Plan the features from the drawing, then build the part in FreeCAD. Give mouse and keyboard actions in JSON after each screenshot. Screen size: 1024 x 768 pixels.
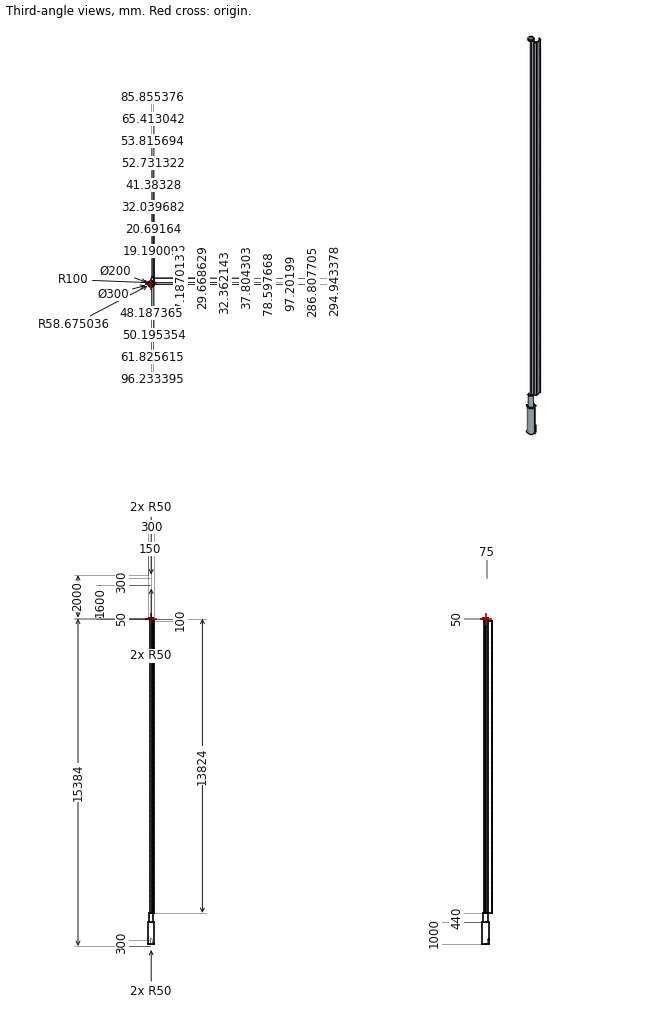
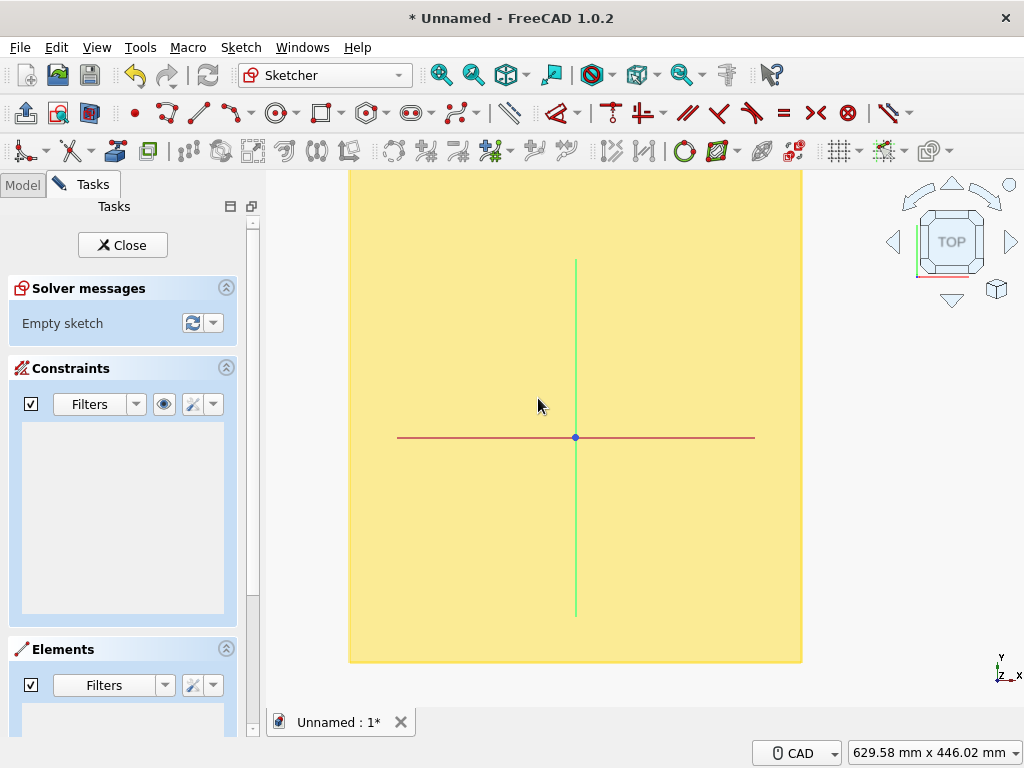
{"action": "left_click", "coordinate": [276, 114]}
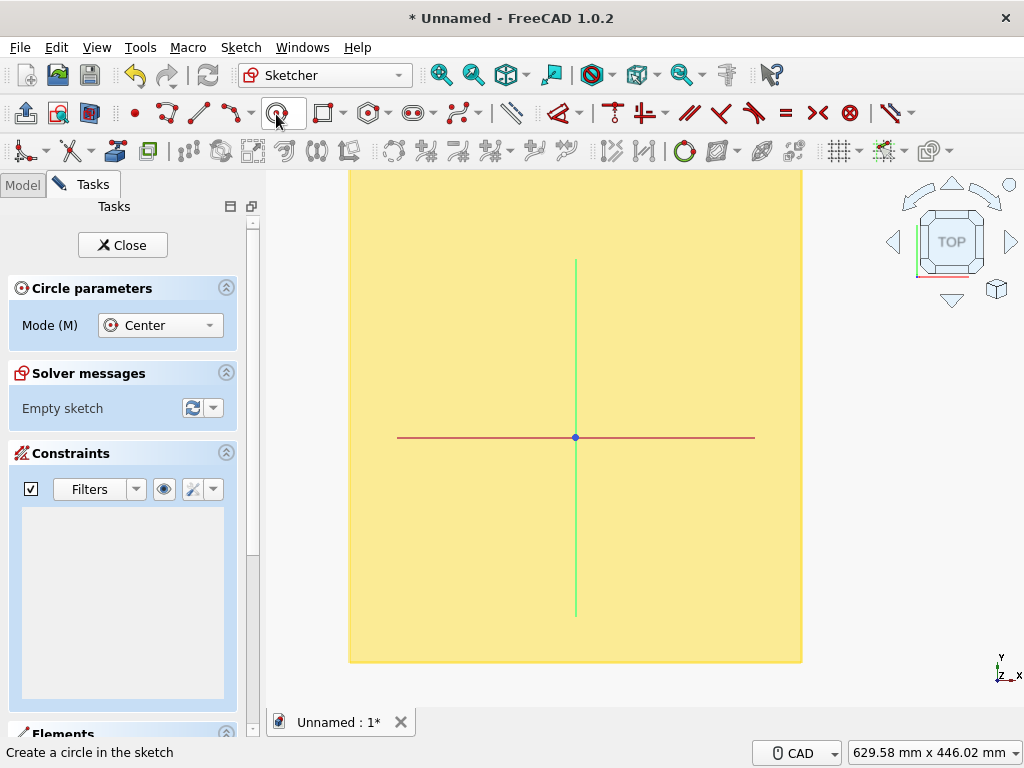
{"action": "left_click", "coordinate": [576, 438]}
{"action": "left_click", "coordinate": [704, 310]}
{"action": "key", "text": "Escape"}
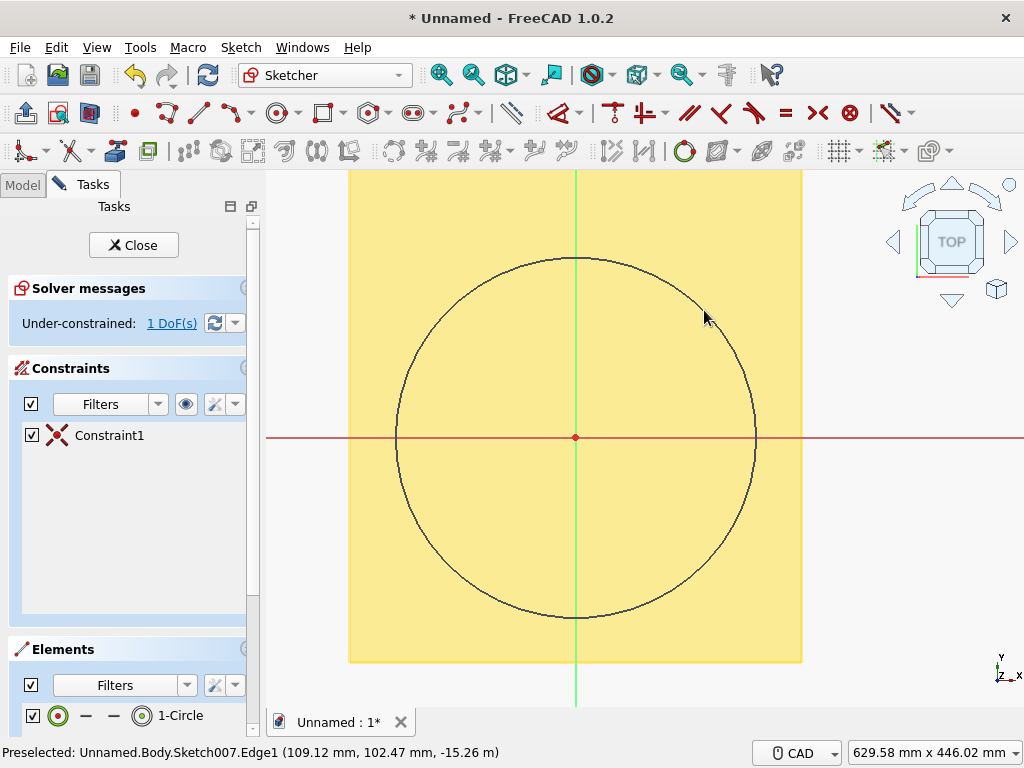
{"action": "left_click", "coordinate": [558, 114]}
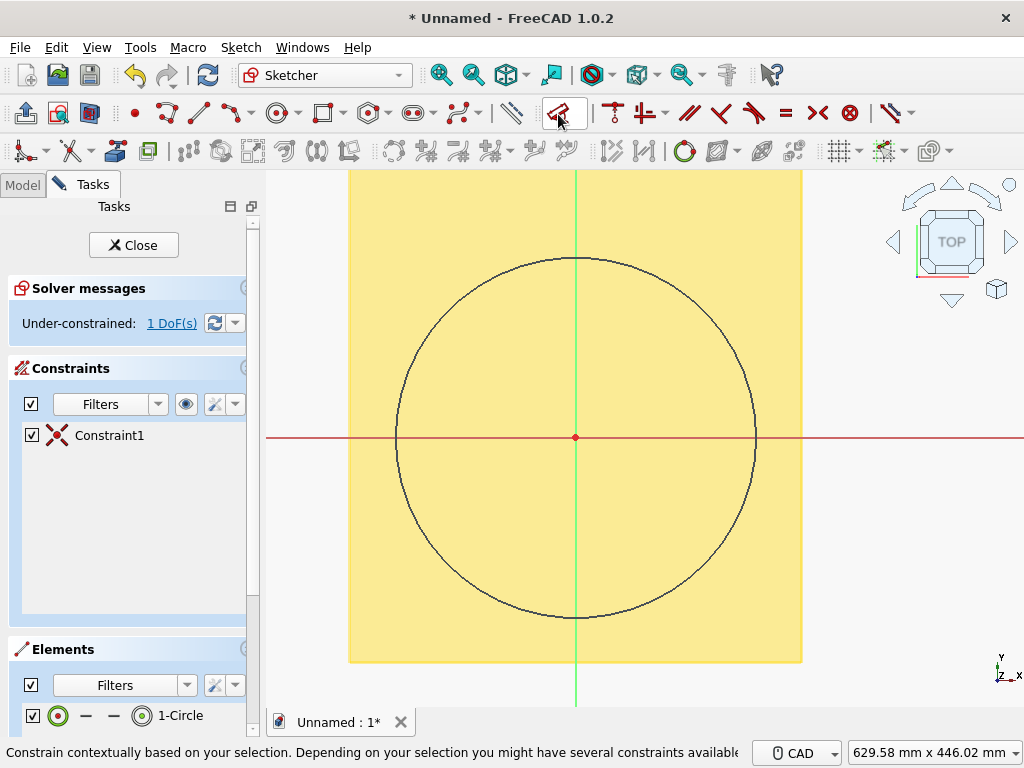
{"action": "left_click", "coordinate": [703, 310]}
{"action": "left_click", "coordinate": [726, 287]}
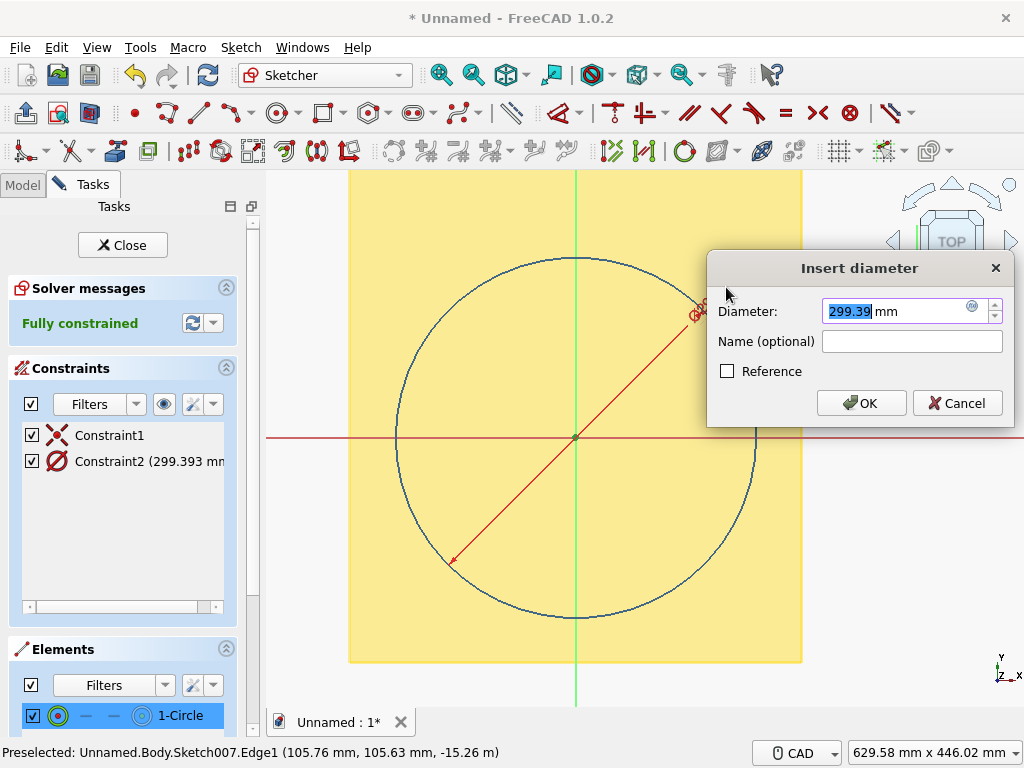
{"action": "type", "text": "300"}
{"action": "key", "text": "Return"}
{"action": "key", "text": "Escape"}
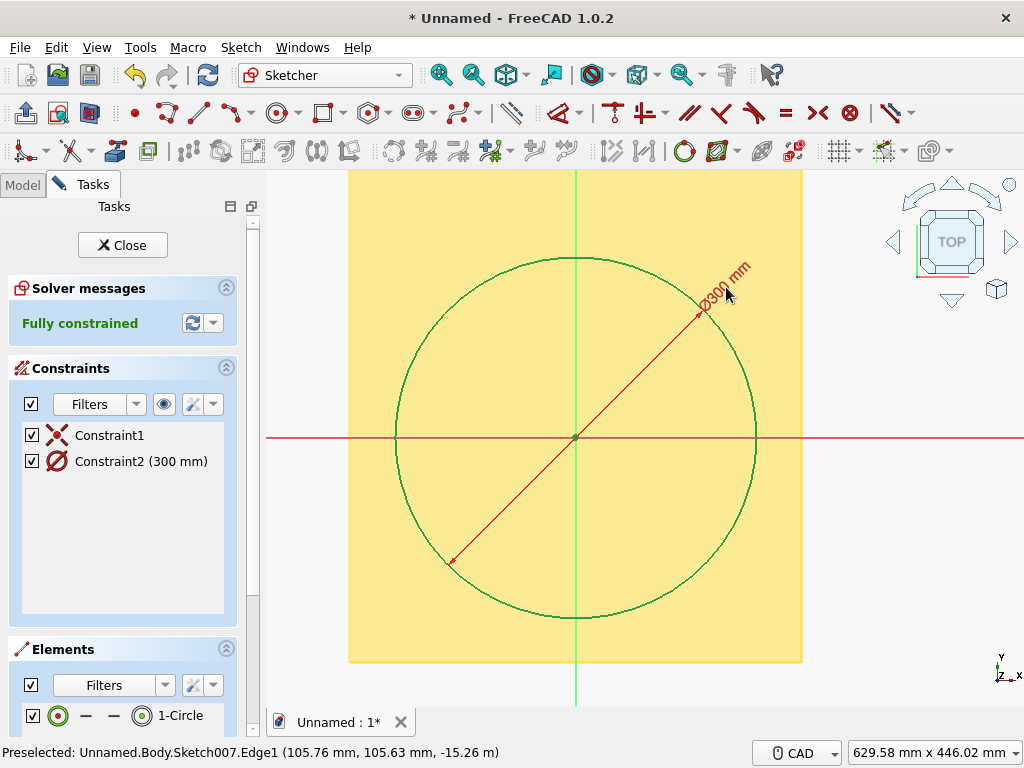
{"action": "left_click", "coordinate": [123, 245]}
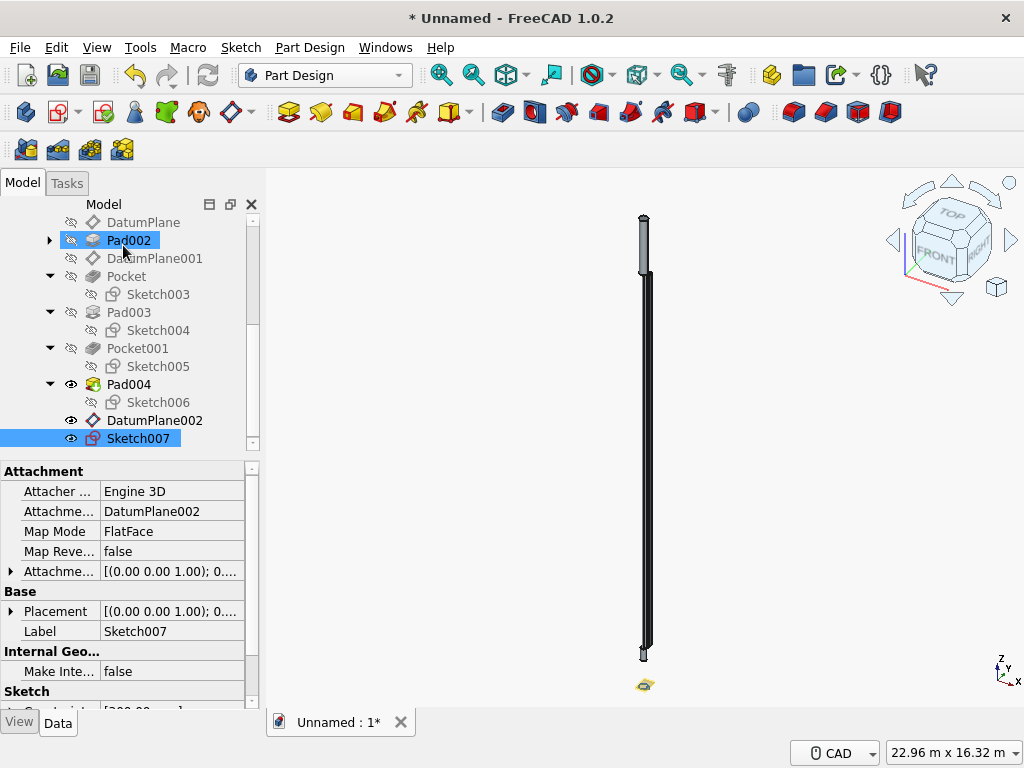
{"action": "left_click", "coordinate": [290, 112]}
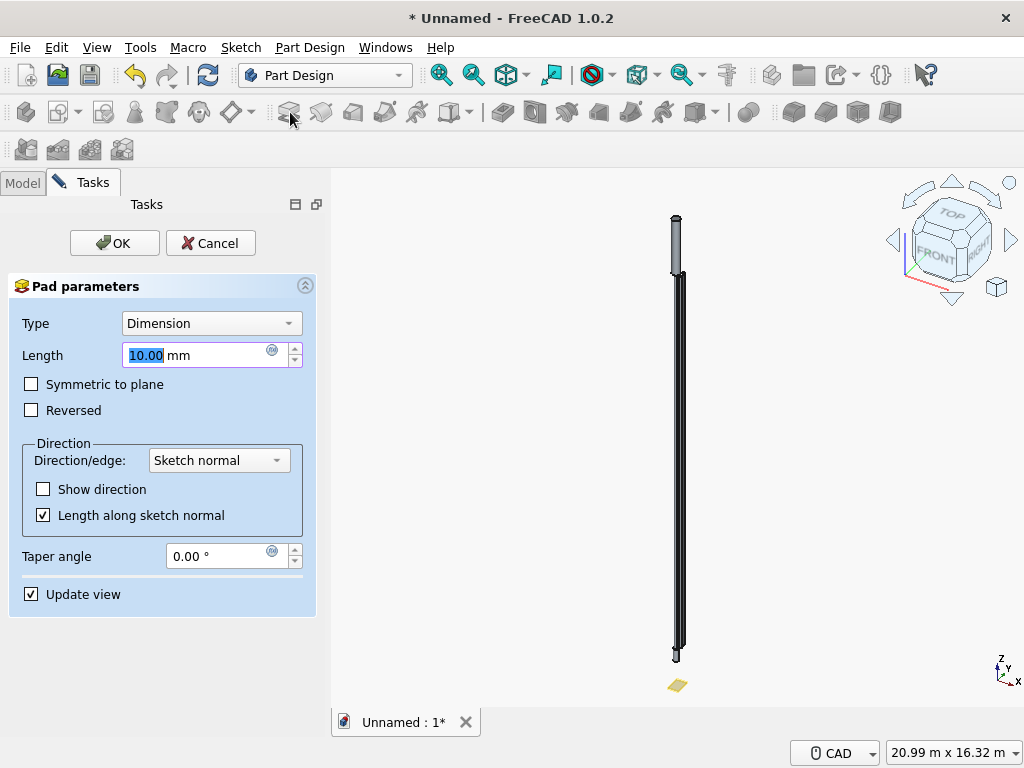
{"action": "type", "text": "1000"}
{"action": "key", "text": "Tab"}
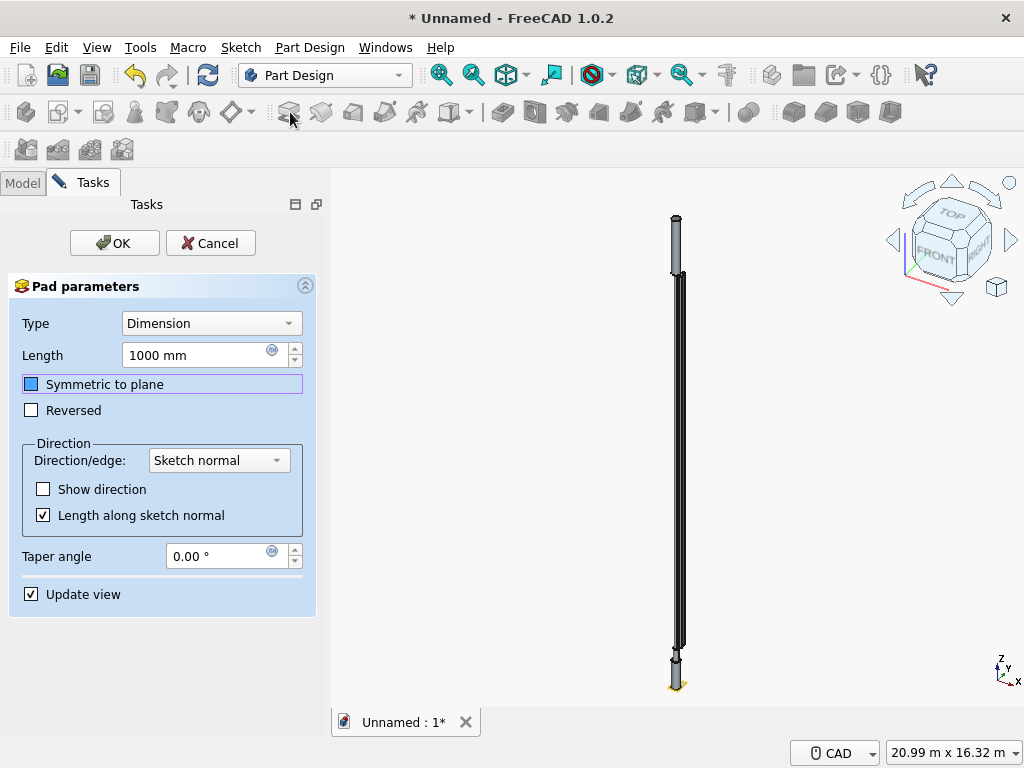
{"action": "left_click", "coordinate": [115, 243]}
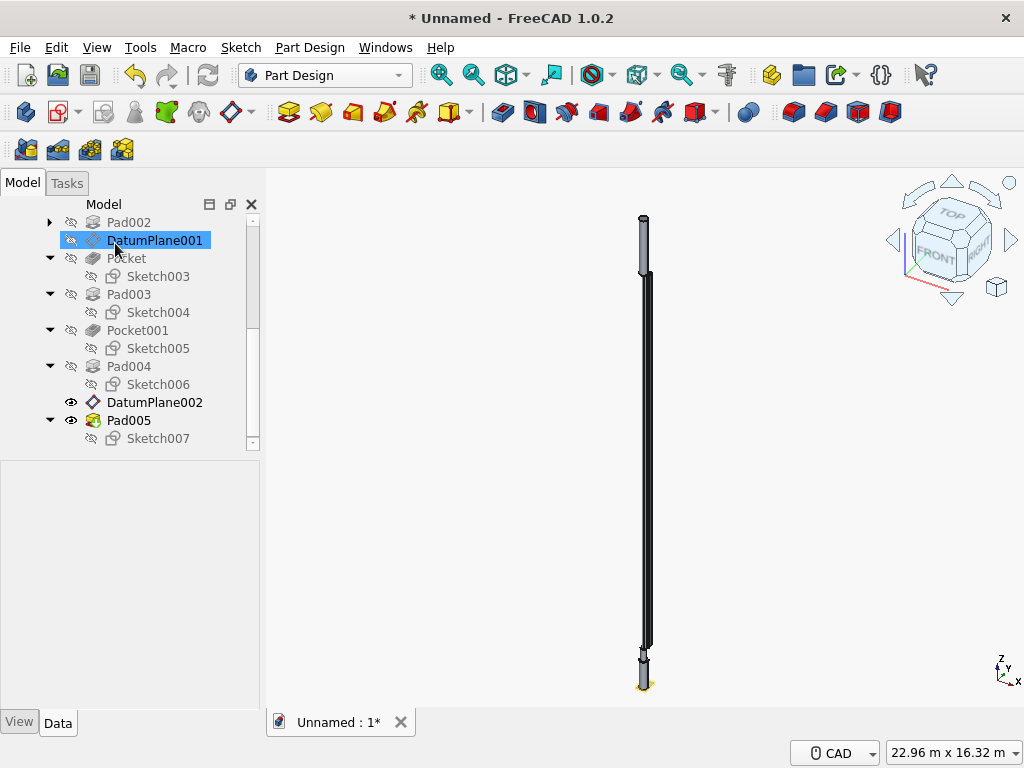
{"action": "left_click", "coordinate": [116, 402]}
{"action": "key", "text": "space"}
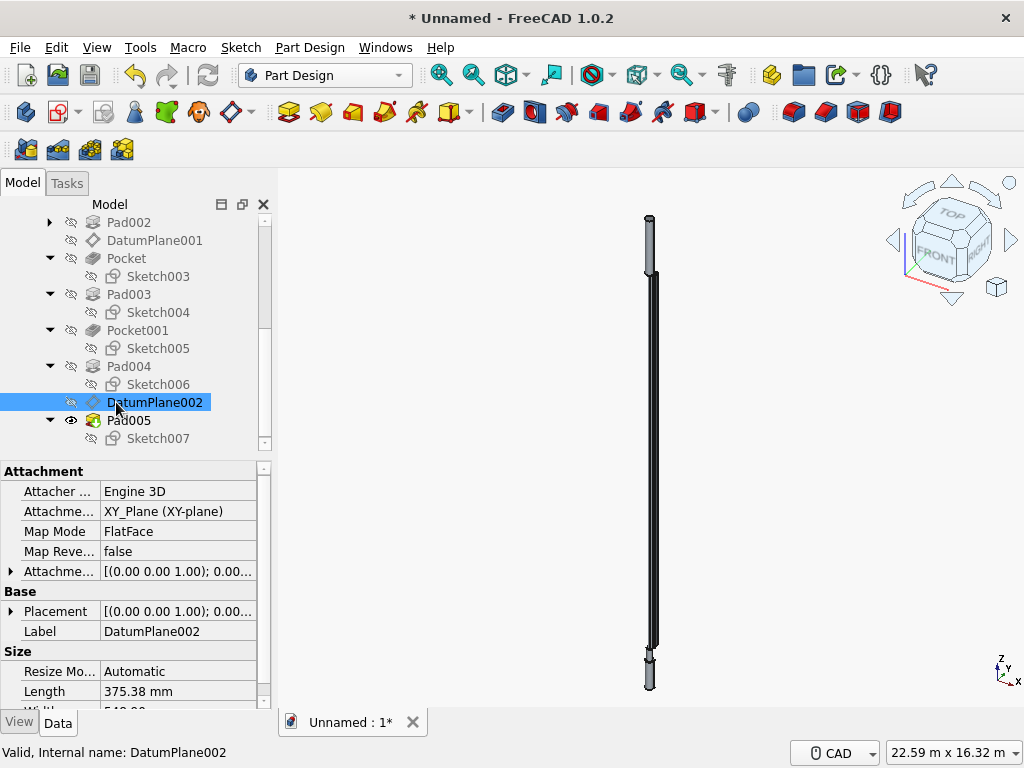
{"action": "scroll", "coordinate": [140, 326], "scroll_direction": "down", "scroll_amount": 3}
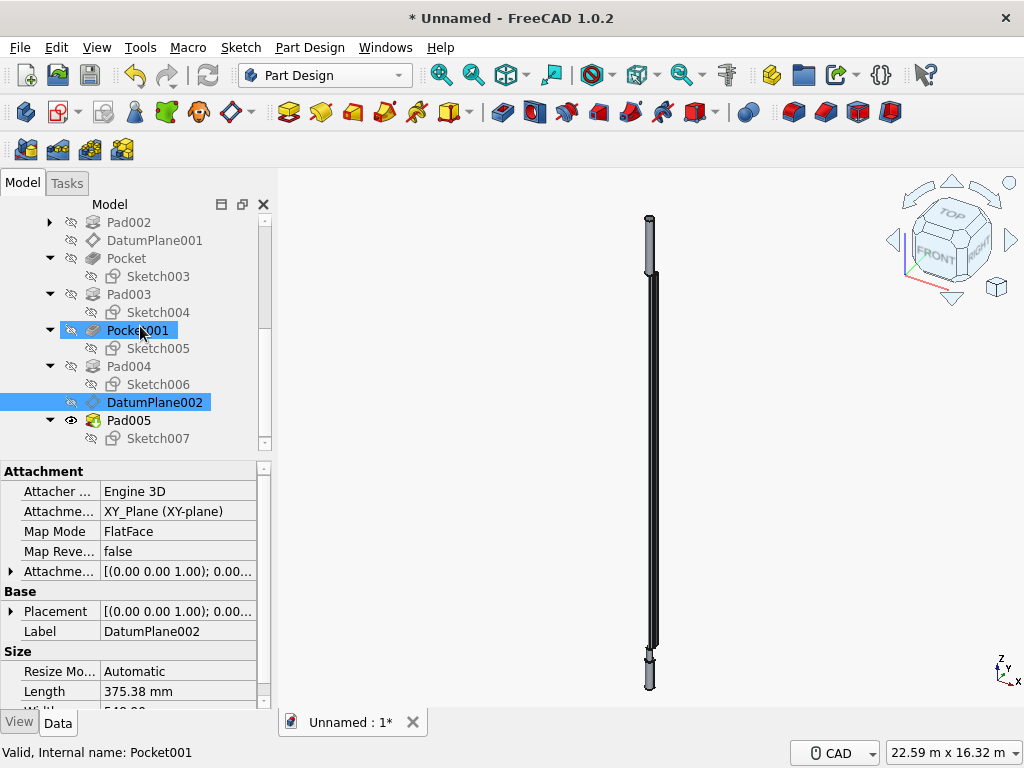
{"action": "scroll", "coordinate": [140, 326], "scroll_direction": "up", "scroll_amount": 15}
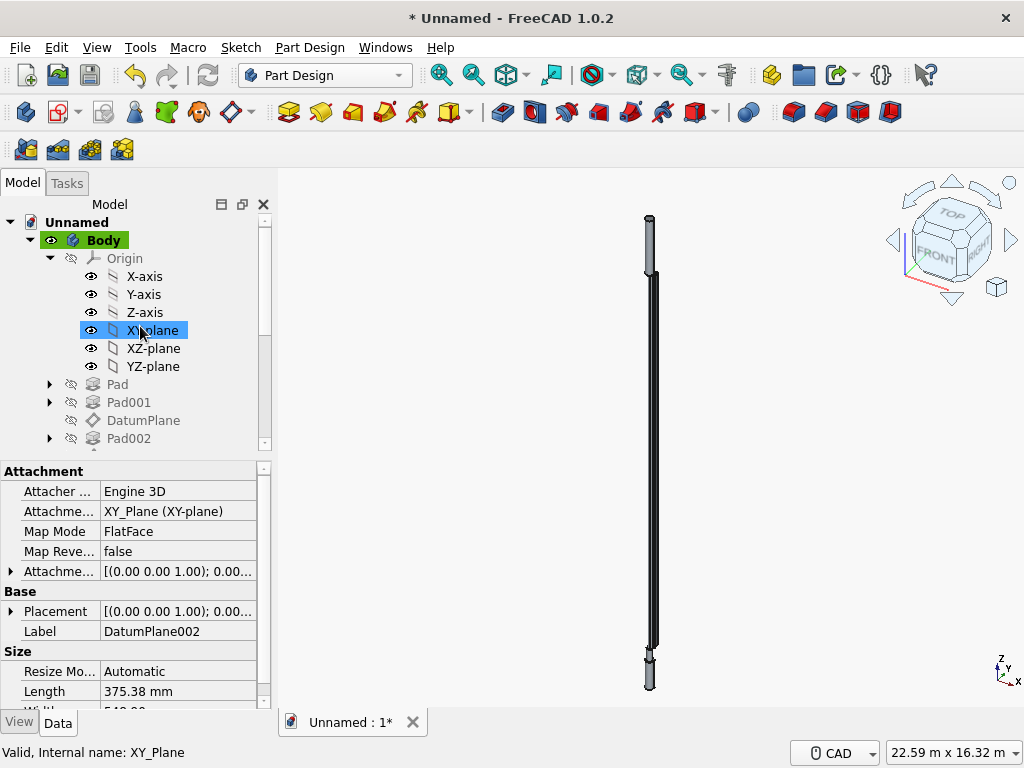
{"action": "left_click", "coordinate": [136, 348]}